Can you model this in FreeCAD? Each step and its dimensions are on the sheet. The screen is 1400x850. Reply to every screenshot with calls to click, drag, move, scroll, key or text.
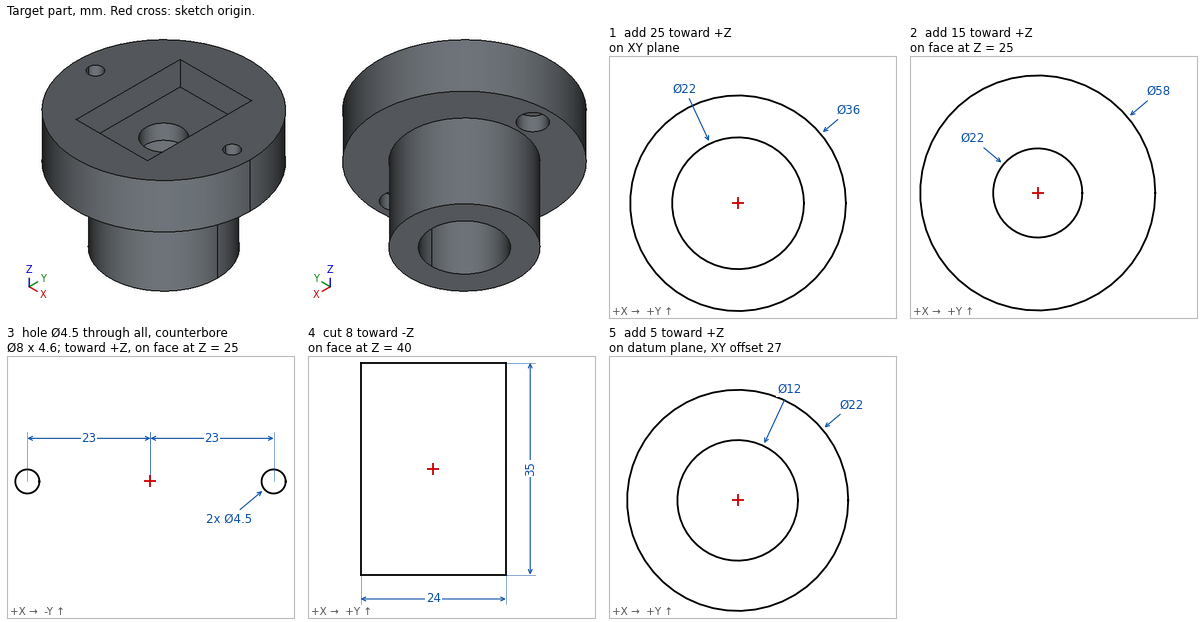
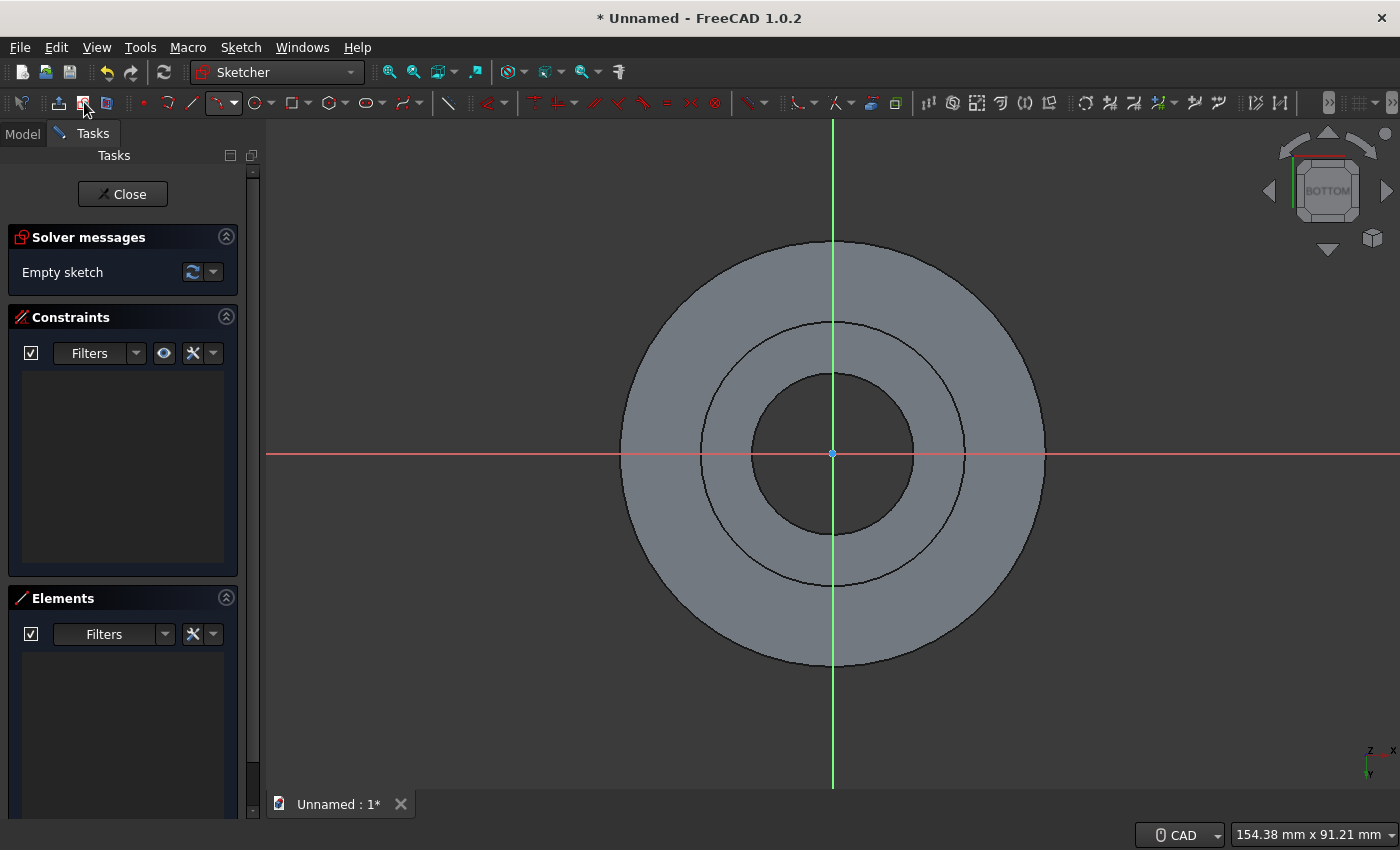
scroll(916, 454, up, 3)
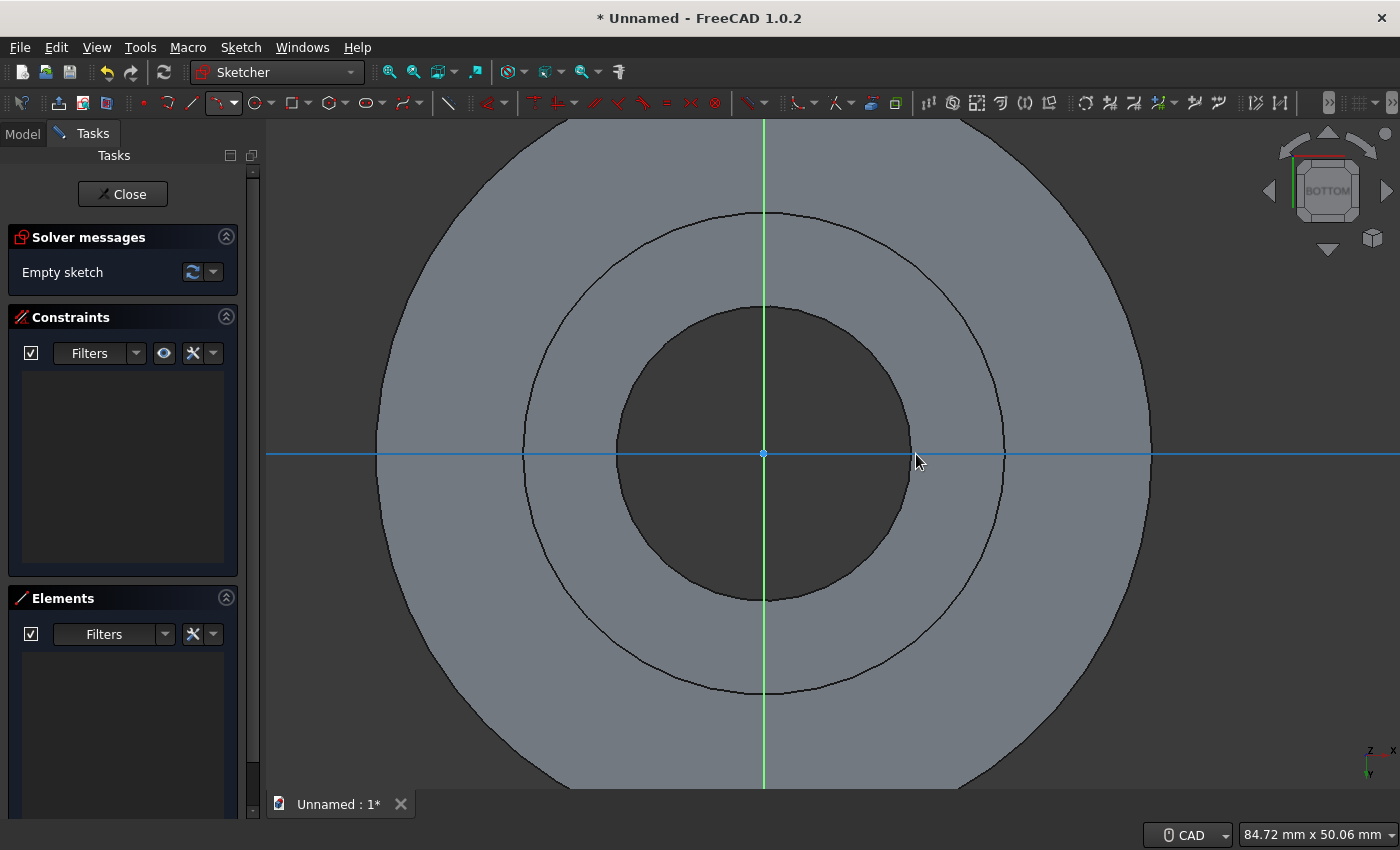
key(g)
key(c)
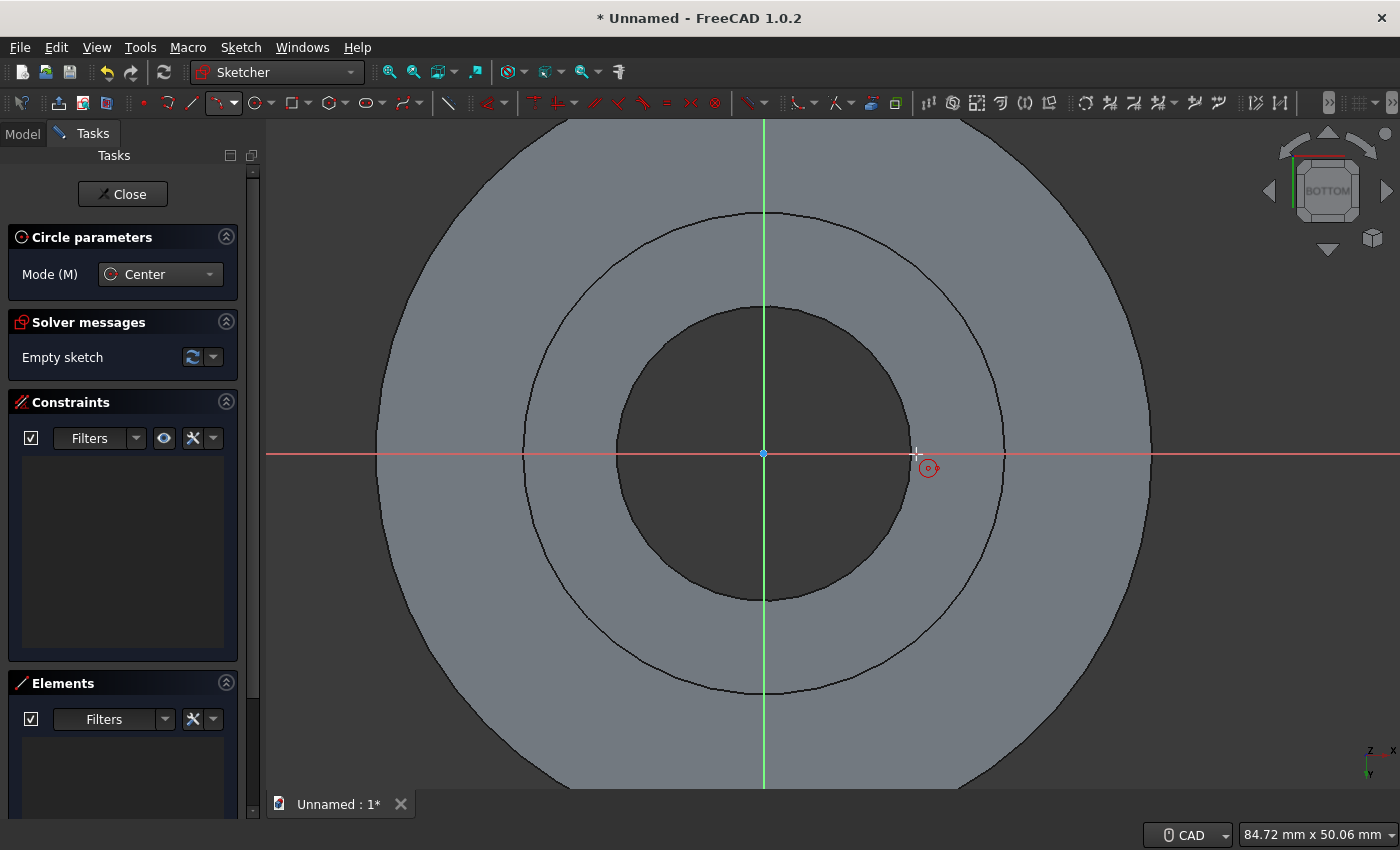
click(1072, 454)
click(1093, 432)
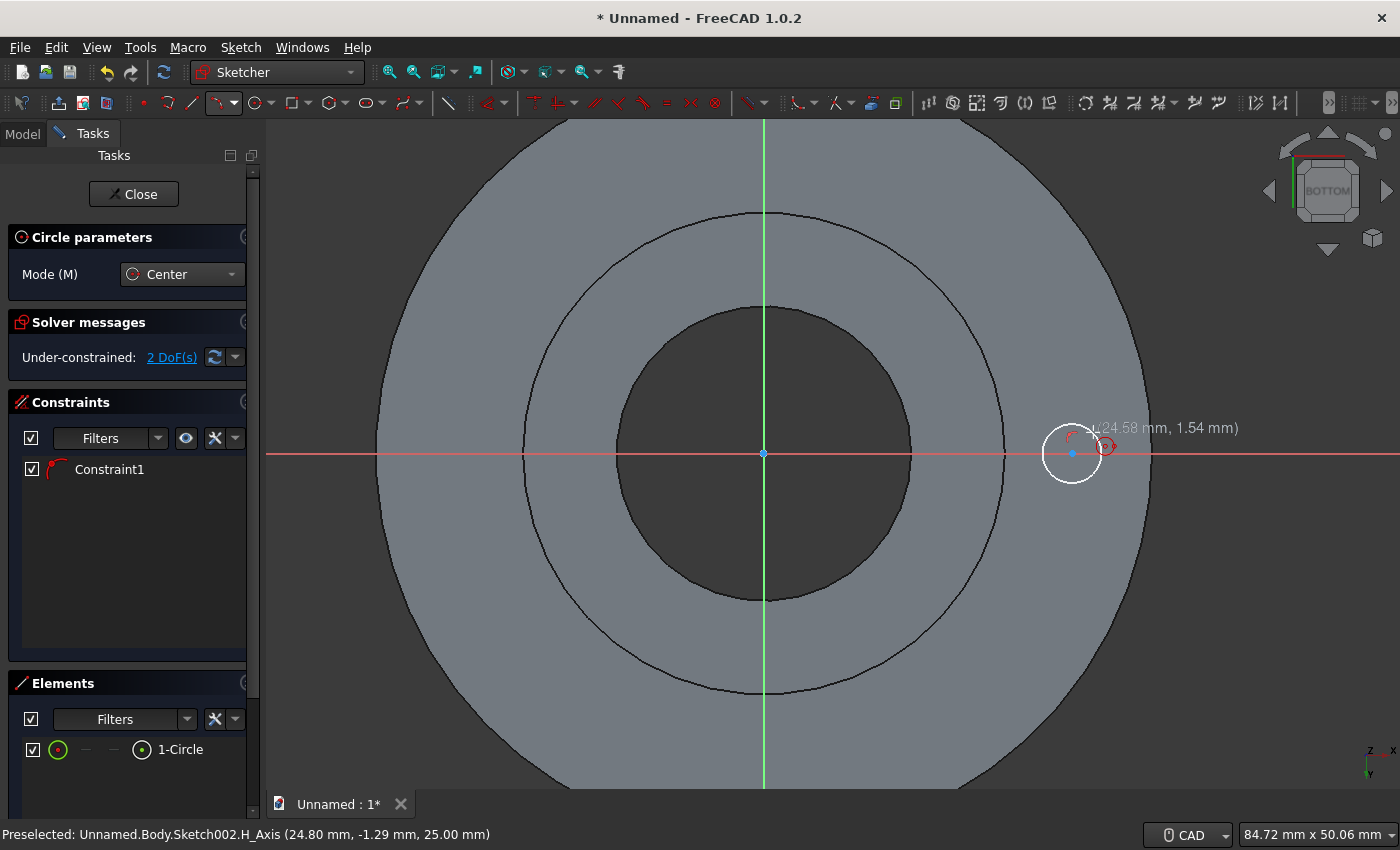
click(456, 454)
click(477, 432)
key(Escape)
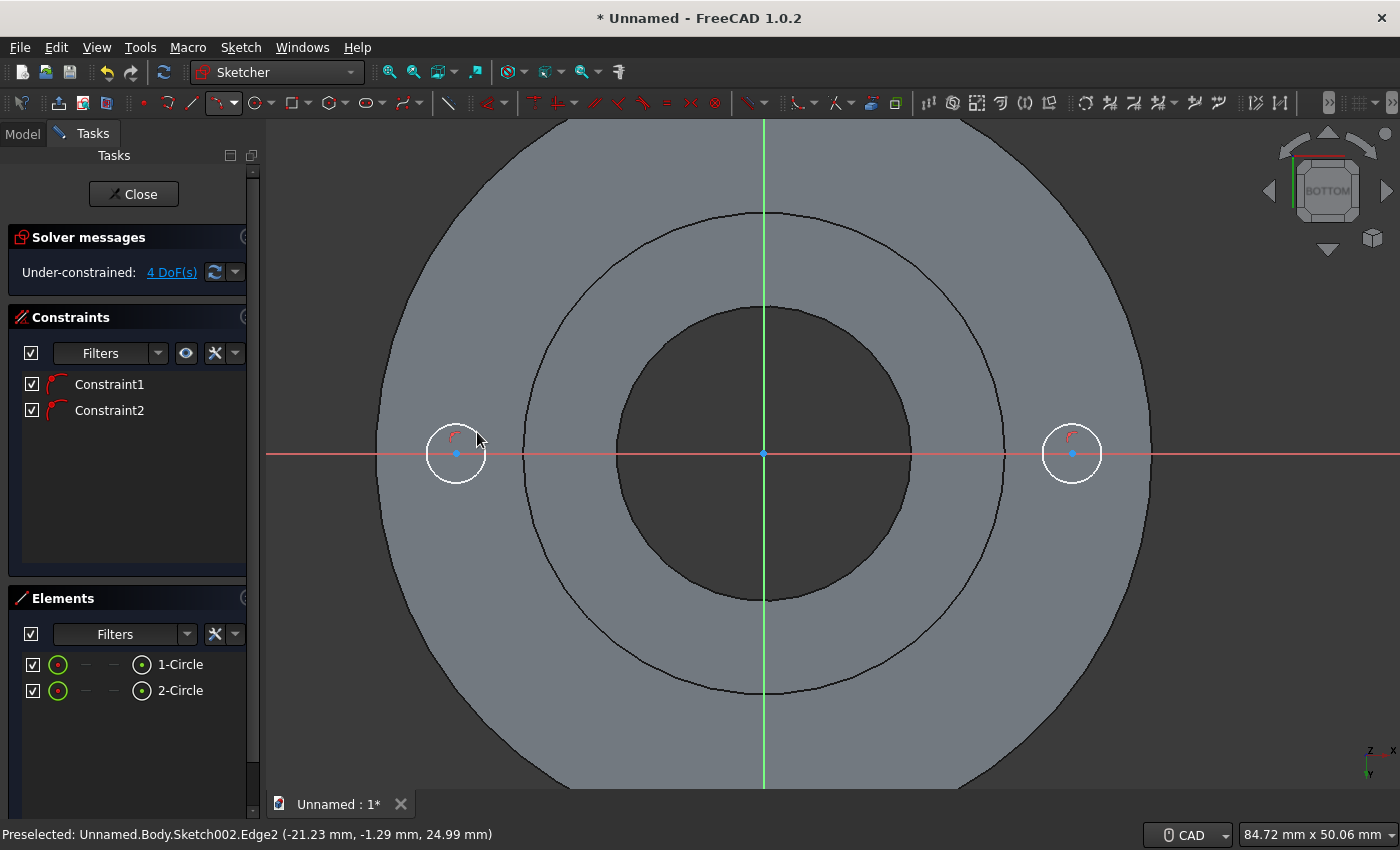
click(1093, 433)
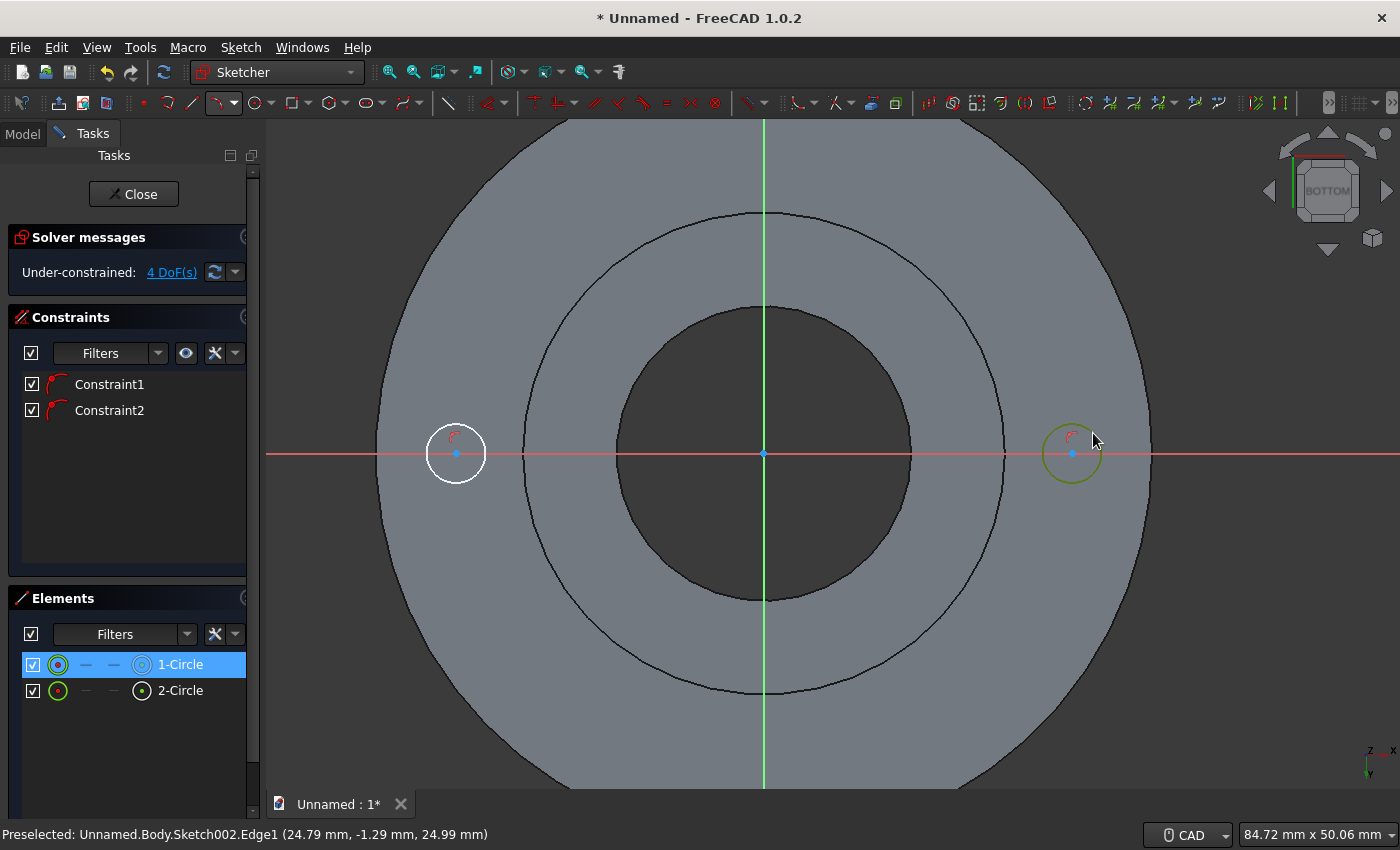
click(477, 433)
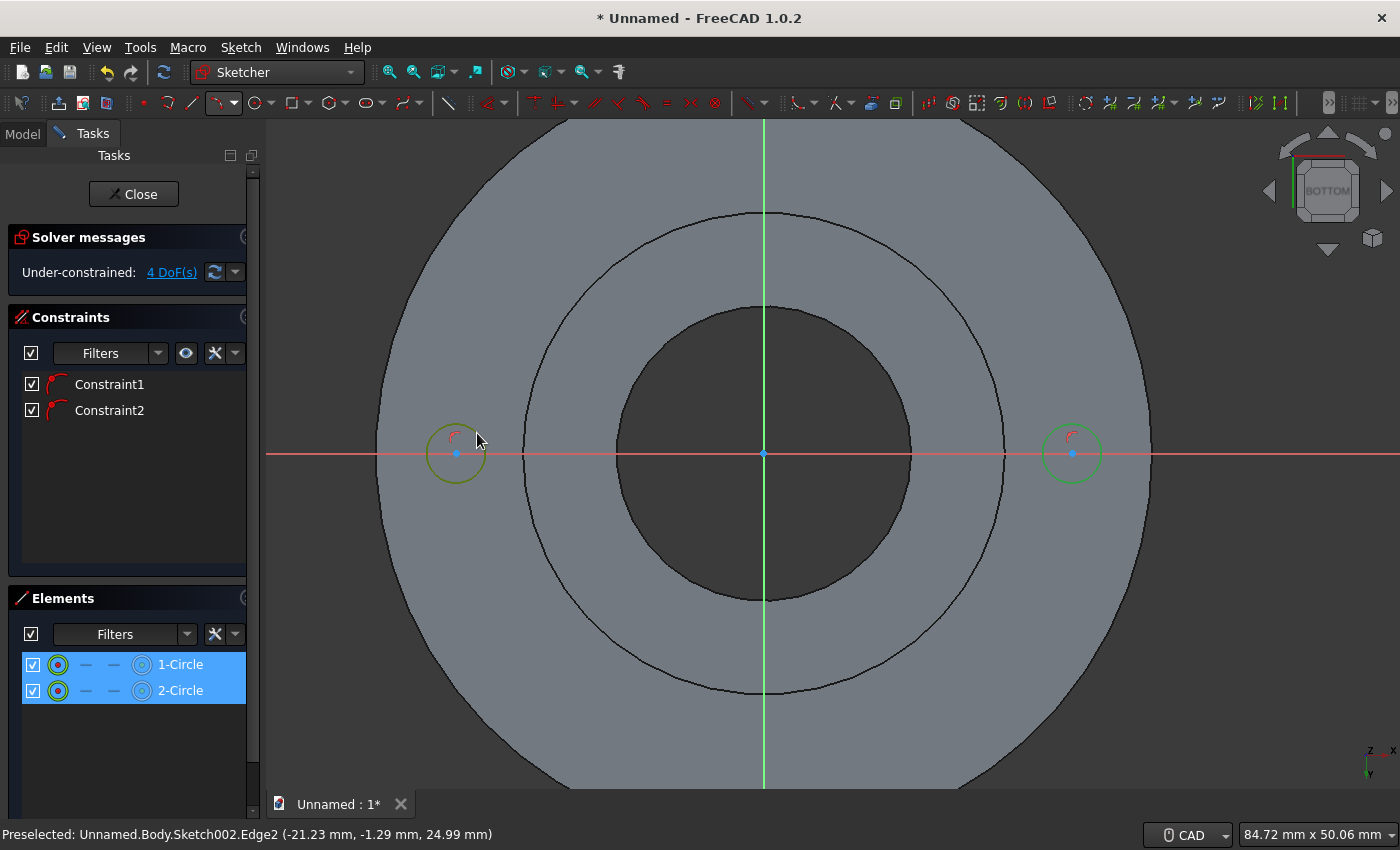
key(e)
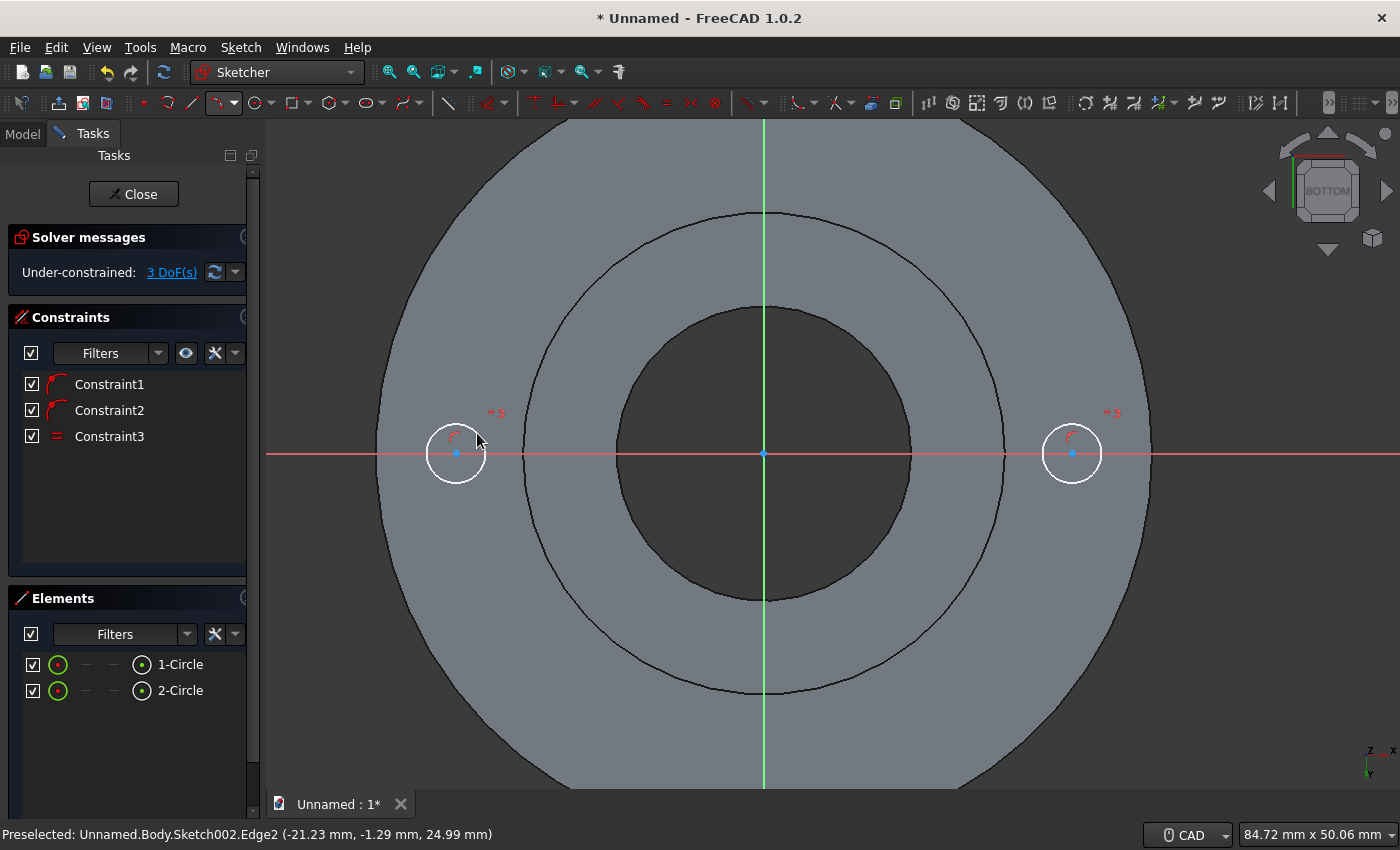
click(488, 104)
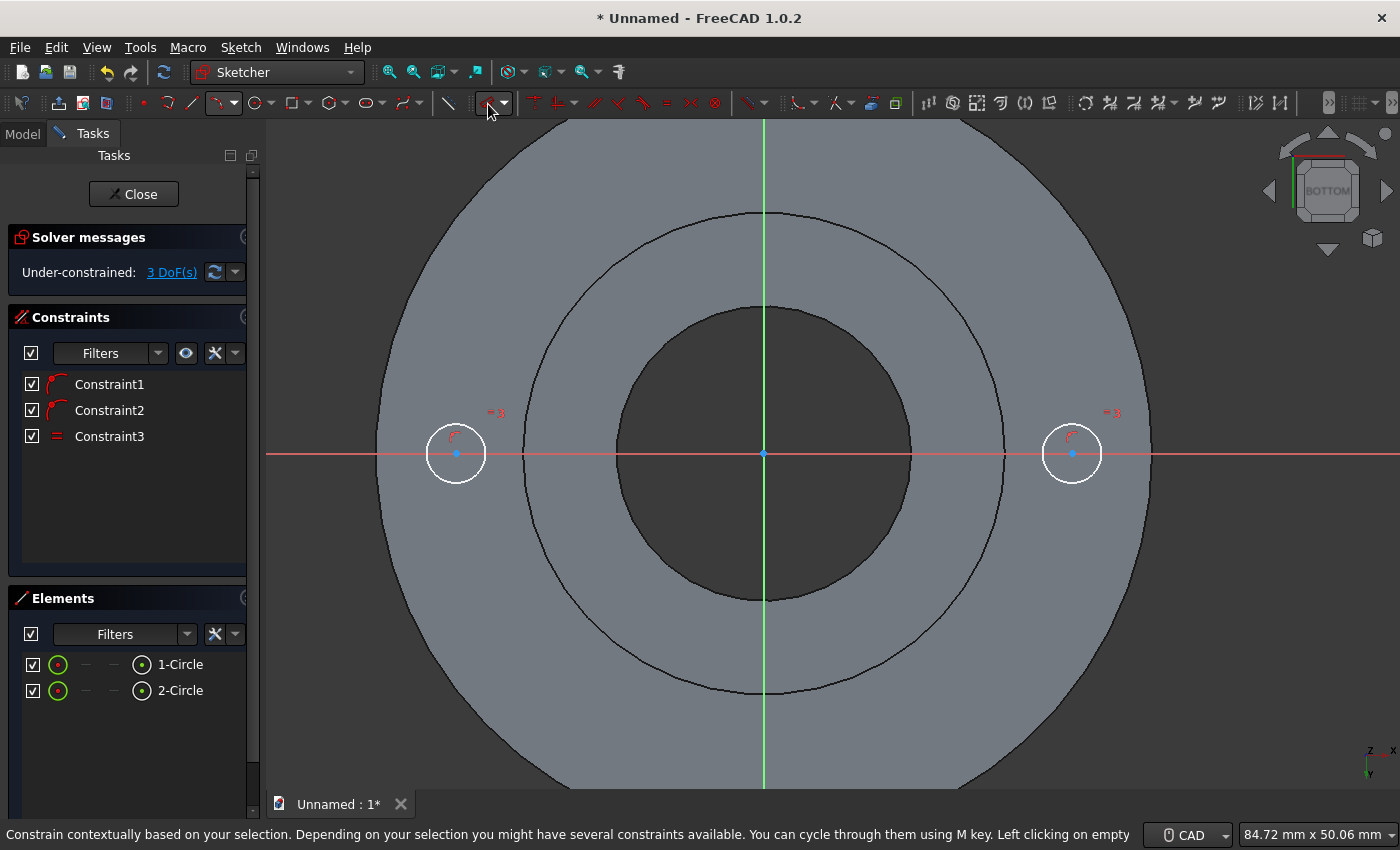
click(1093, 433)
click(1116, 411)